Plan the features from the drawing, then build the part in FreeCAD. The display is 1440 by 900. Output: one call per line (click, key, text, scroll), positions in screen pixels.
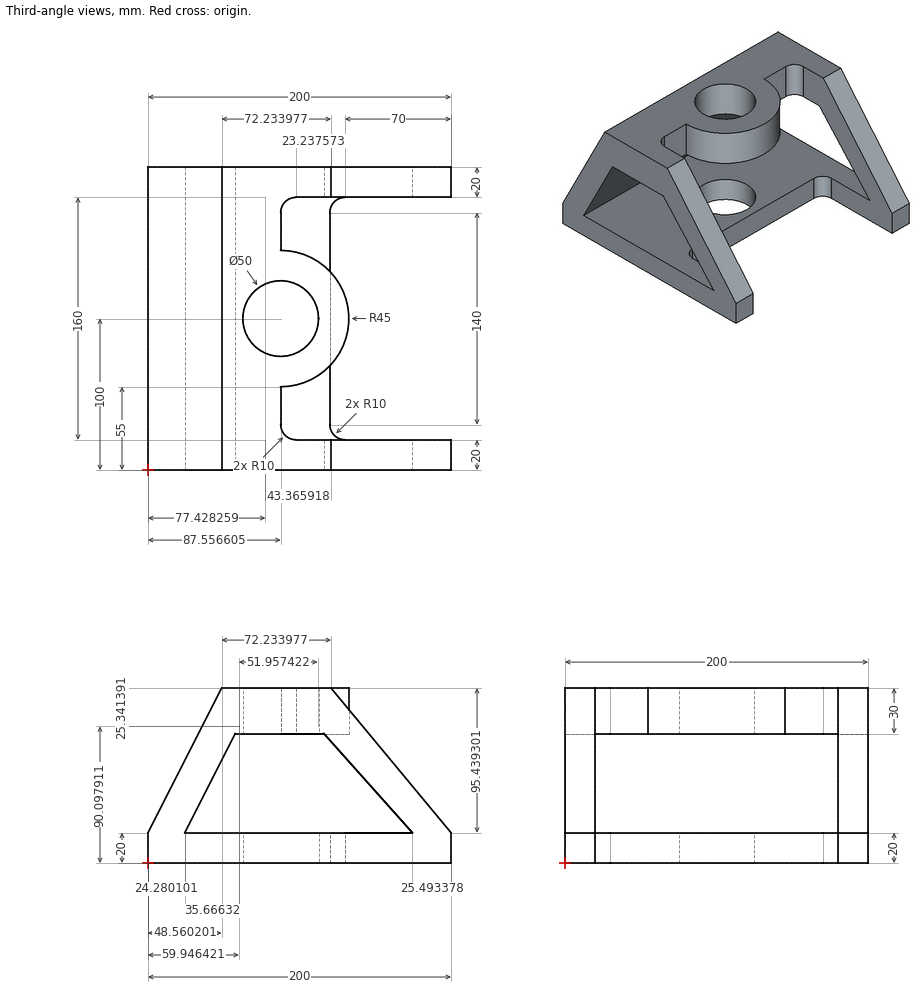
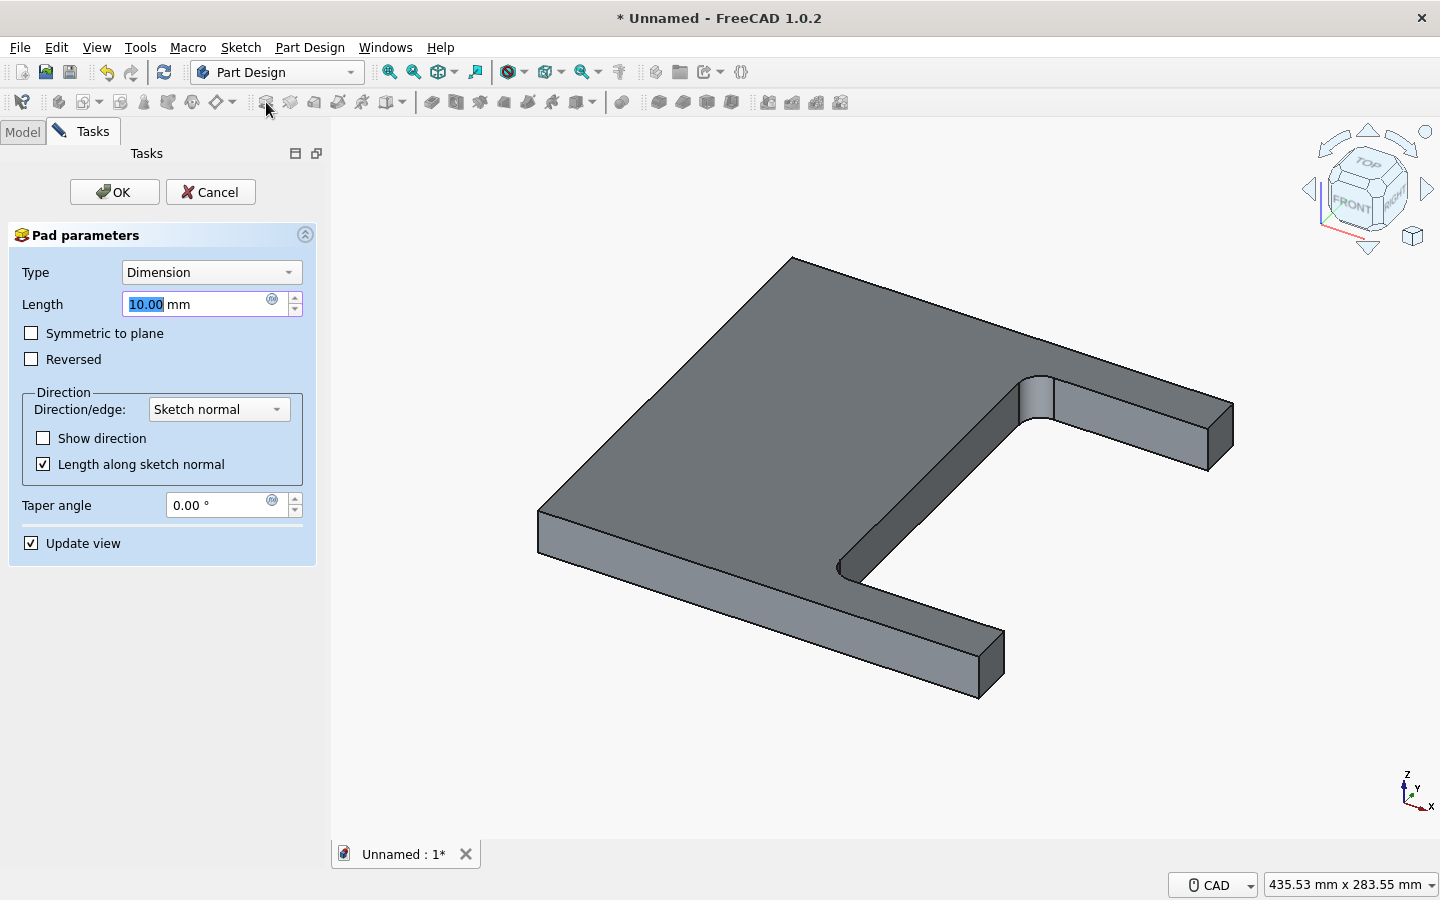
text(200)
key(Tab)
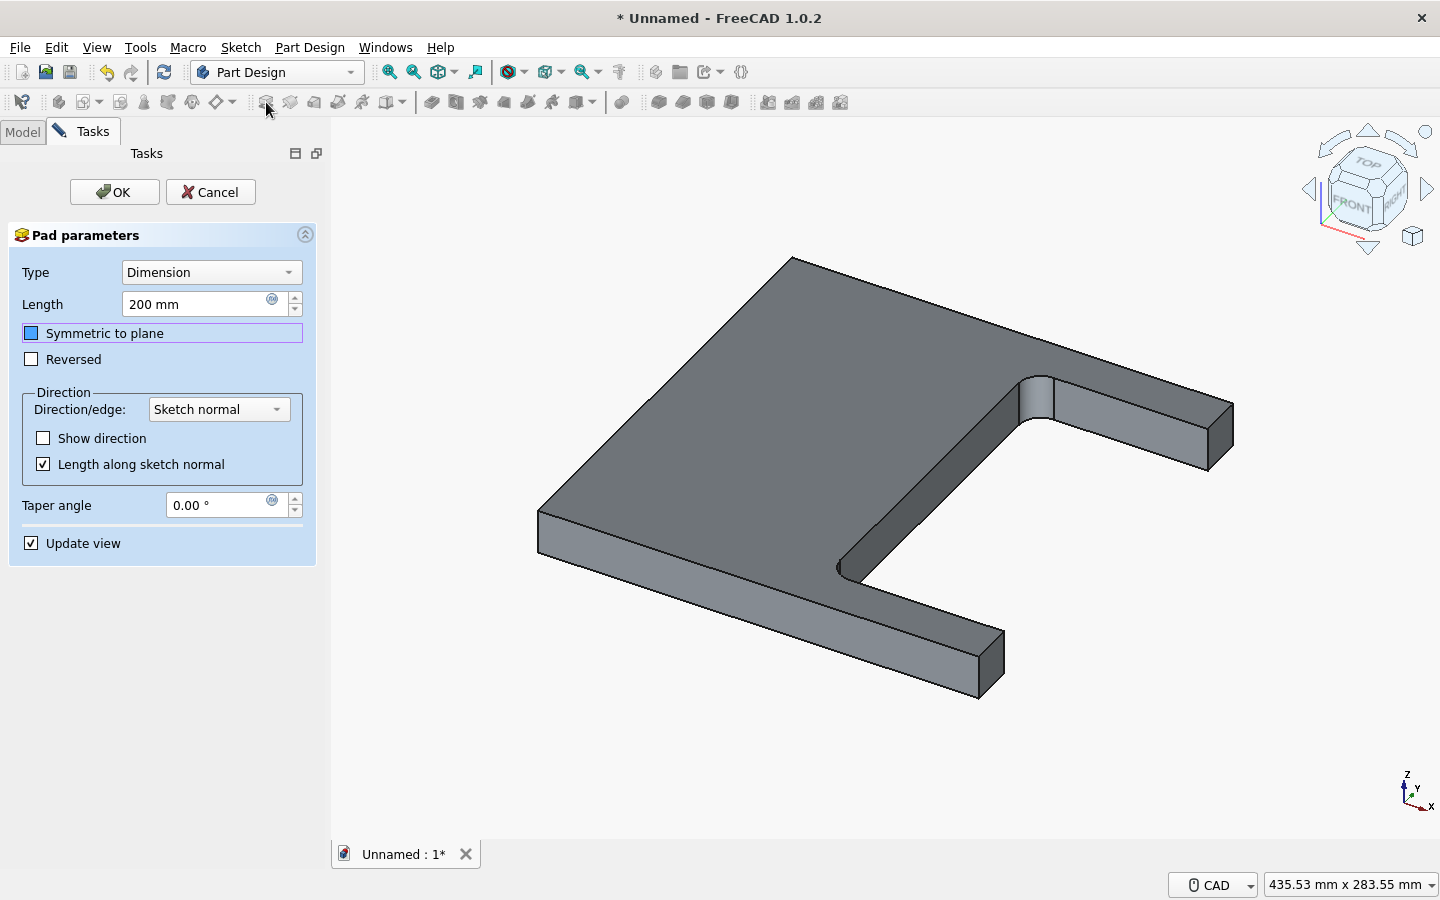
click(30, 359)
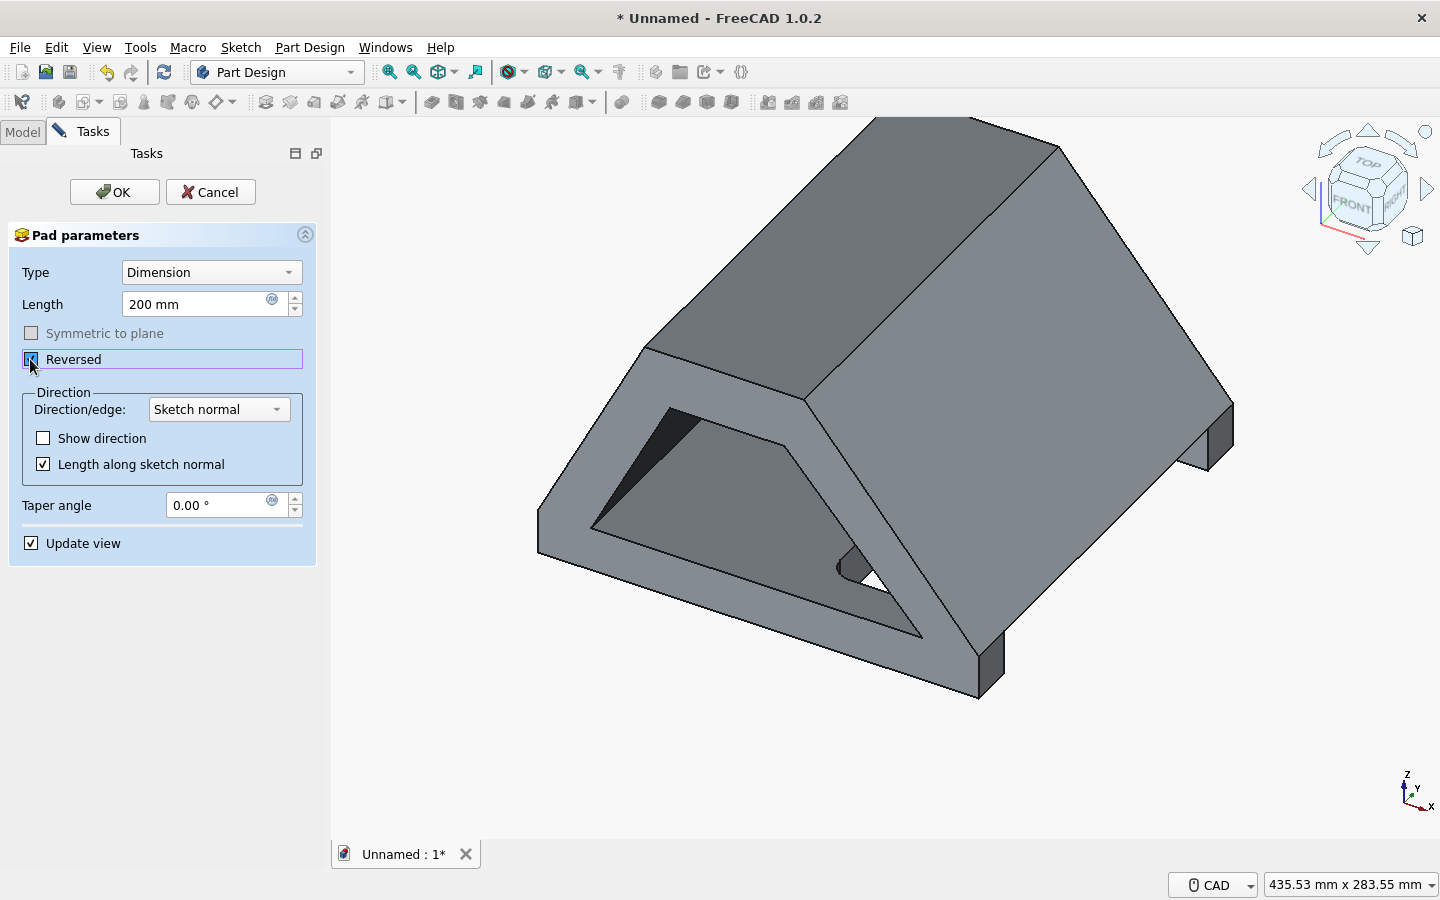
click(115, 192)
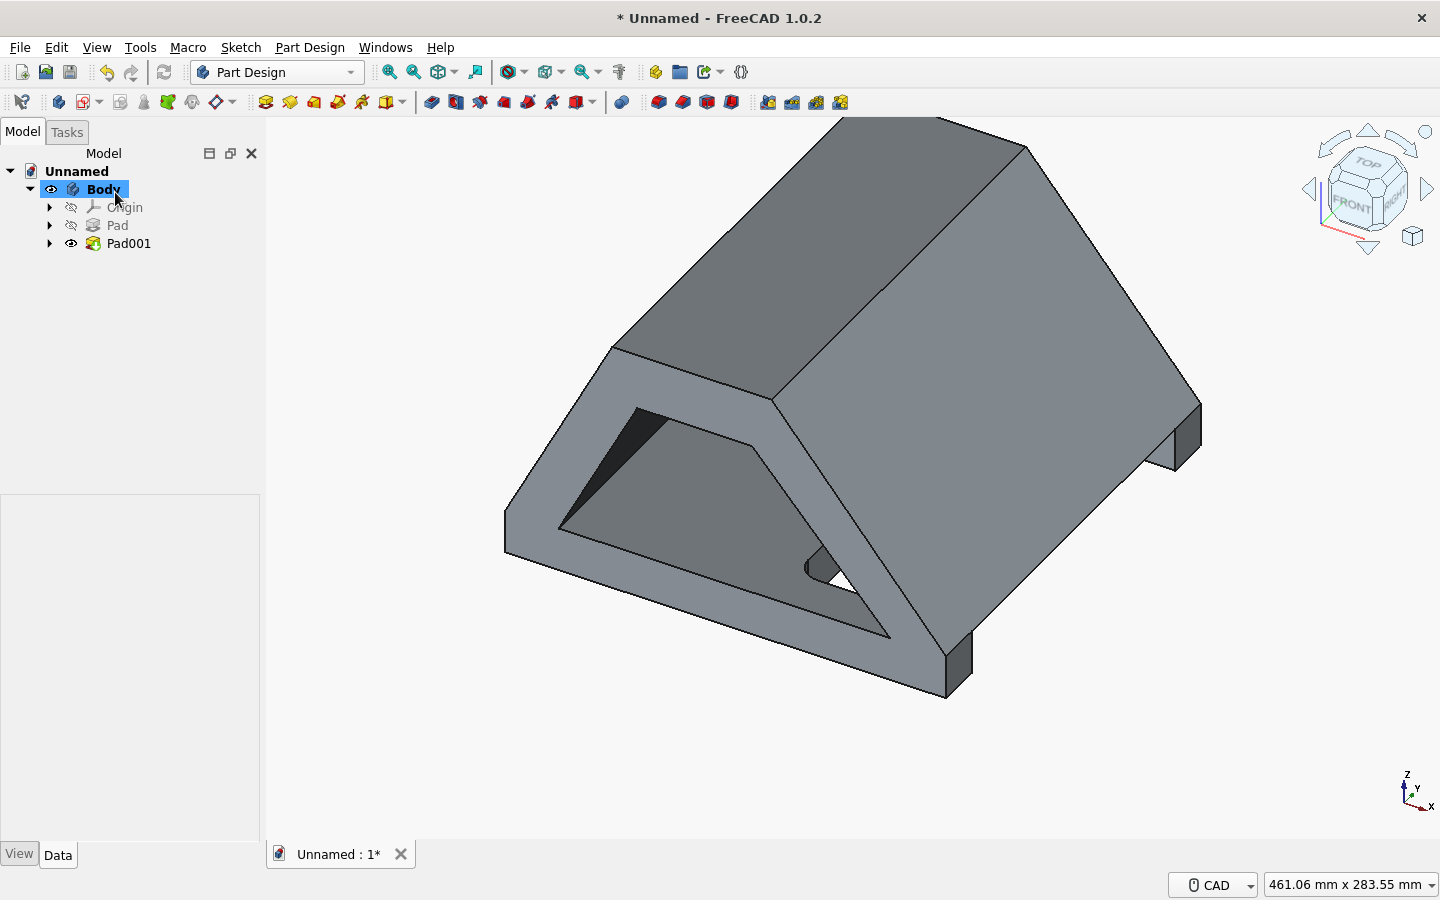
click(390, 72)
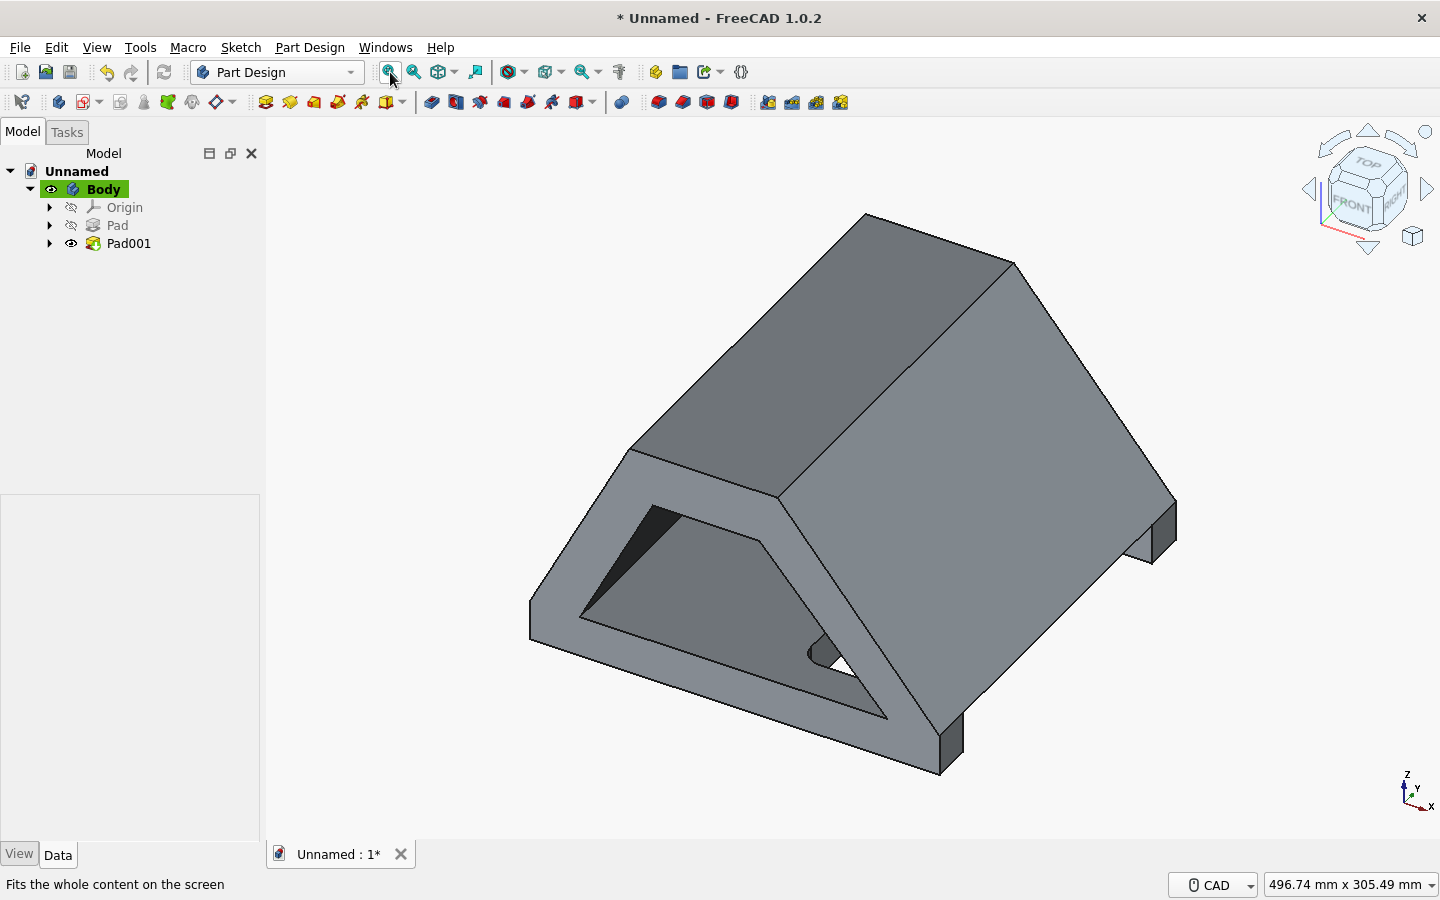
click(1010, 465)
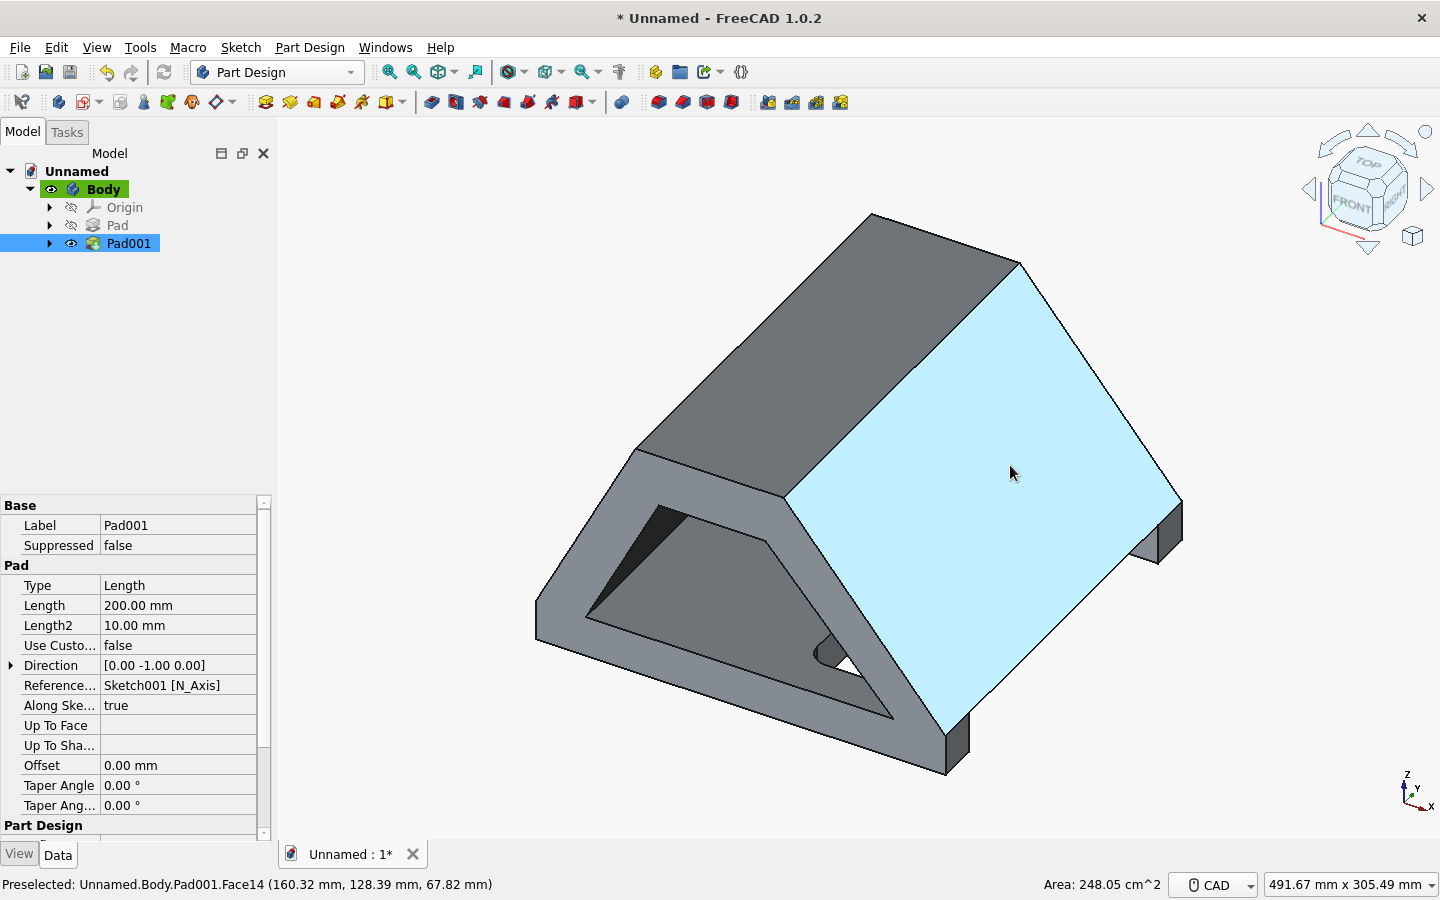
click(84, 102)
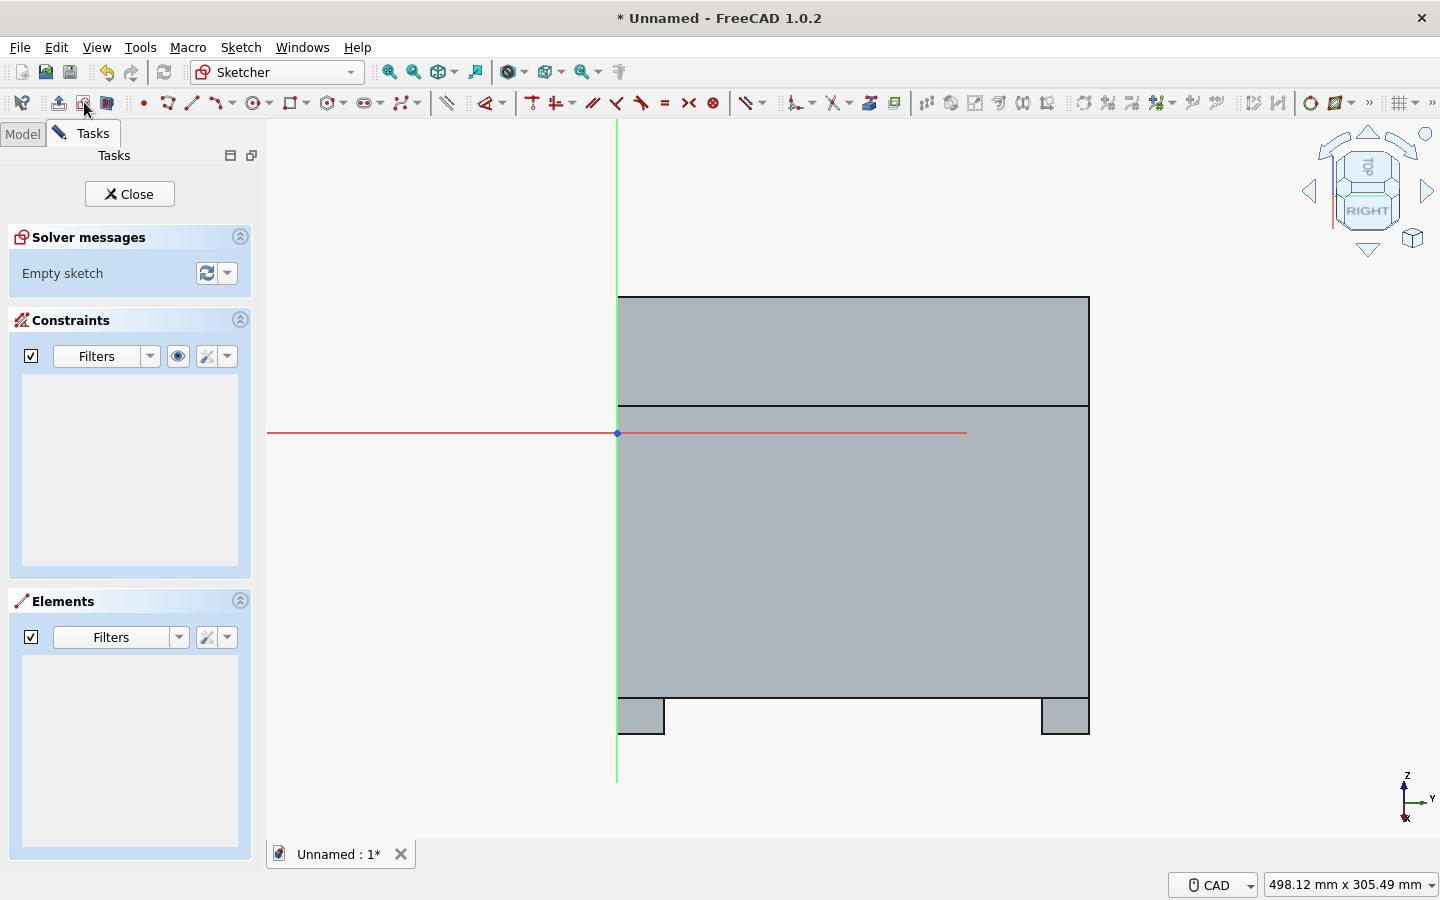
scroll(921, 700, up, 2)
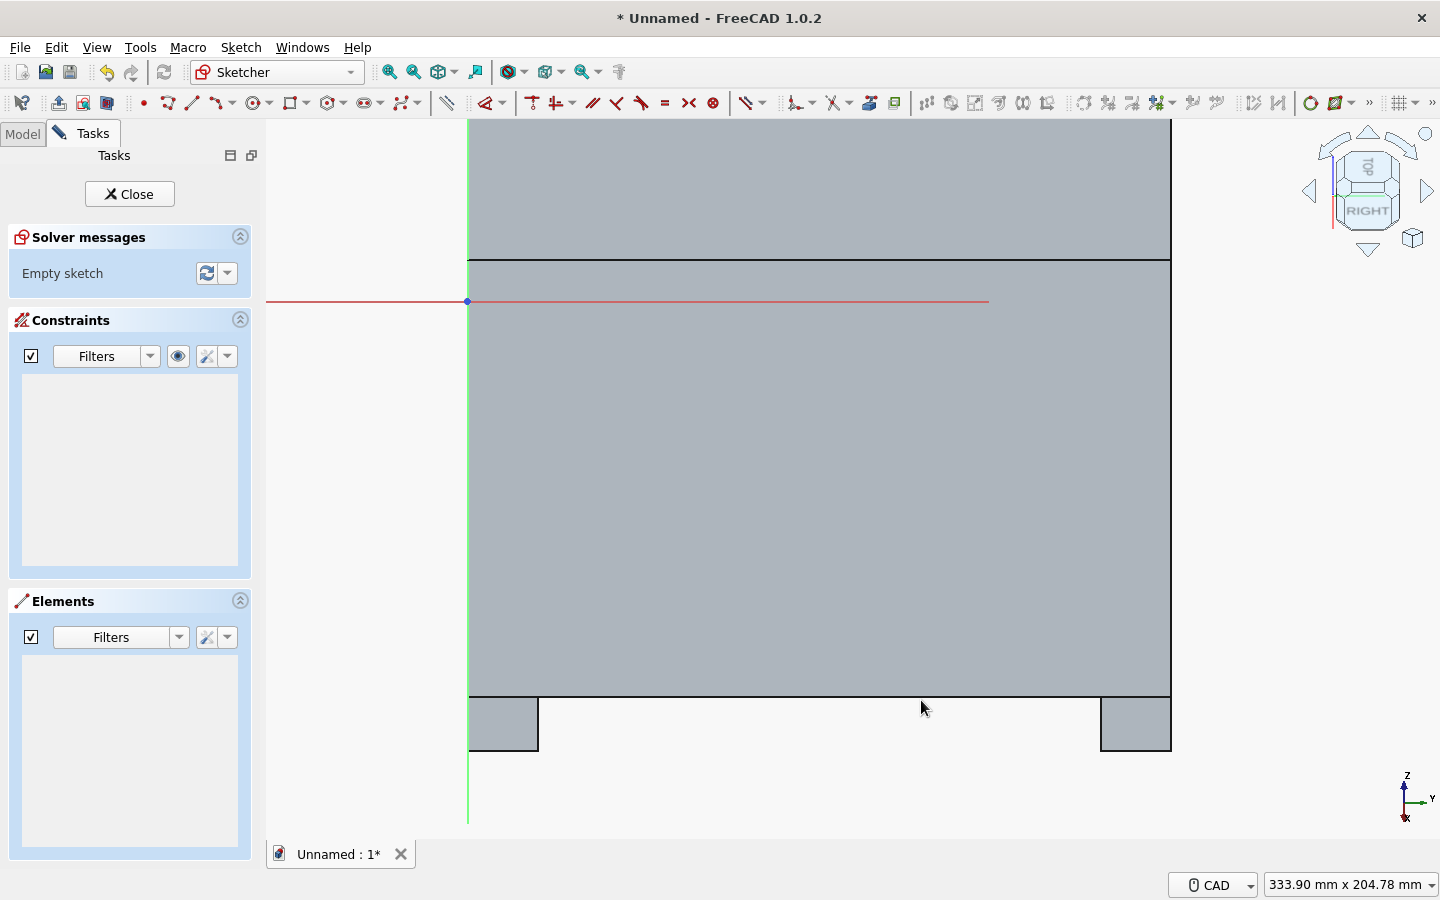
click(290, 104)